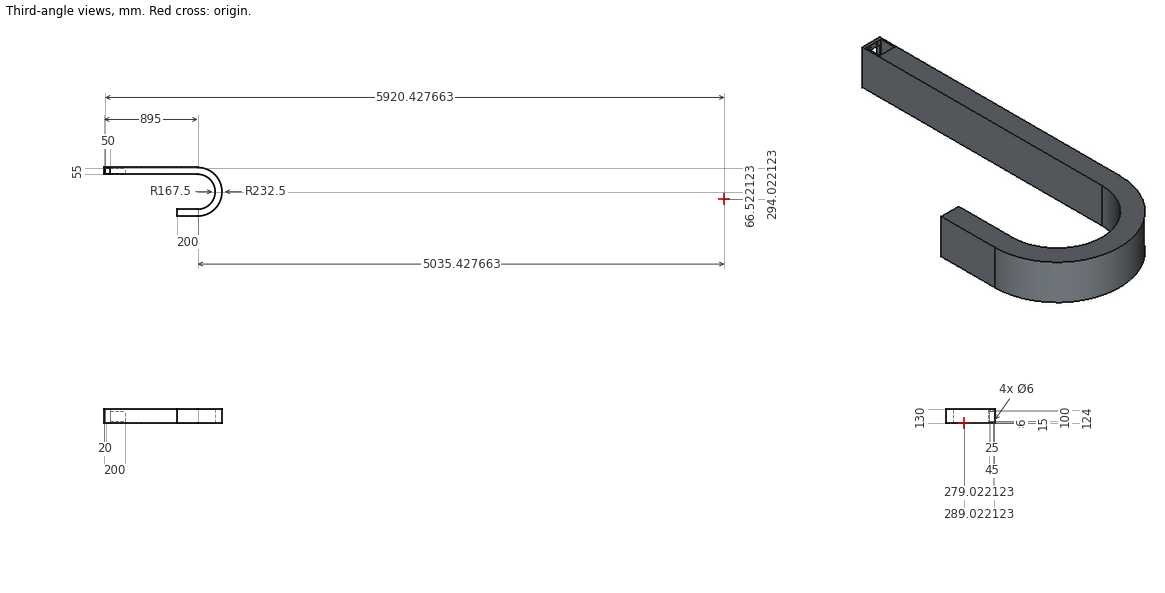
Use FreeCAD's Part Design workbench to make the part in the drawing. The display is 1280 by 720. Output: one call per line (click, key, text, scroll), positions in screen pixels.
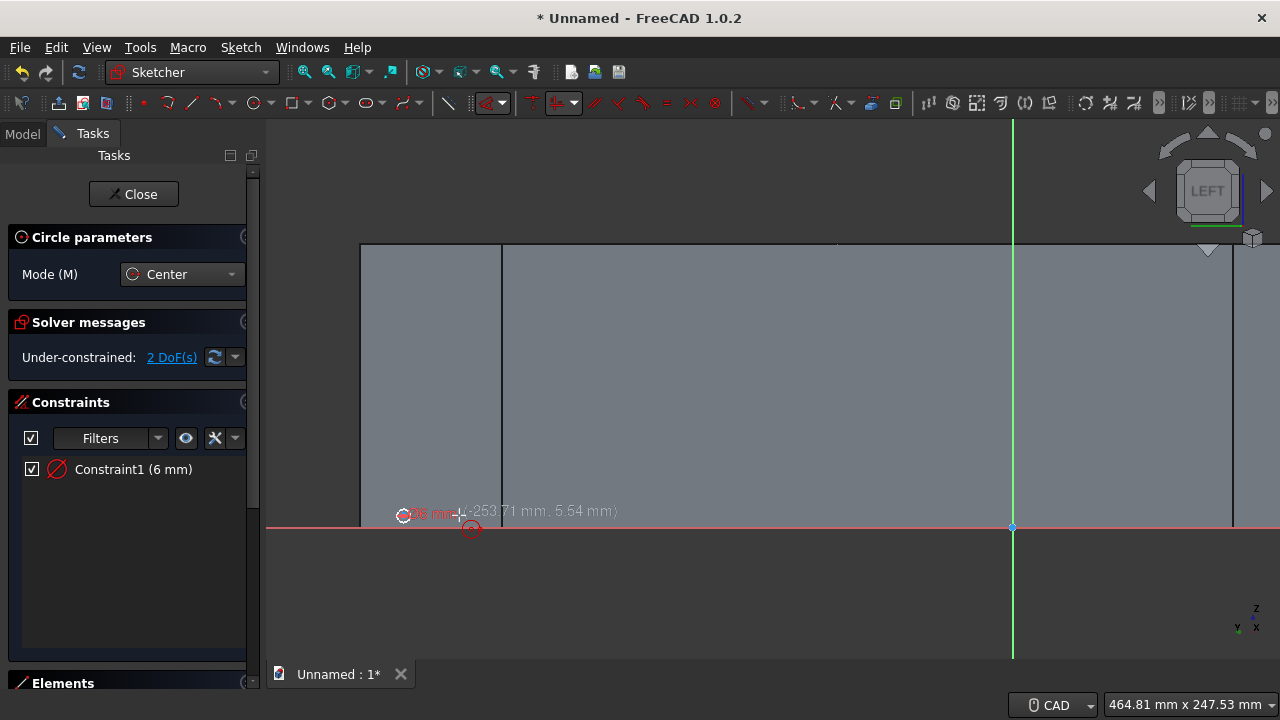
click(458, 515)
move(463, 510)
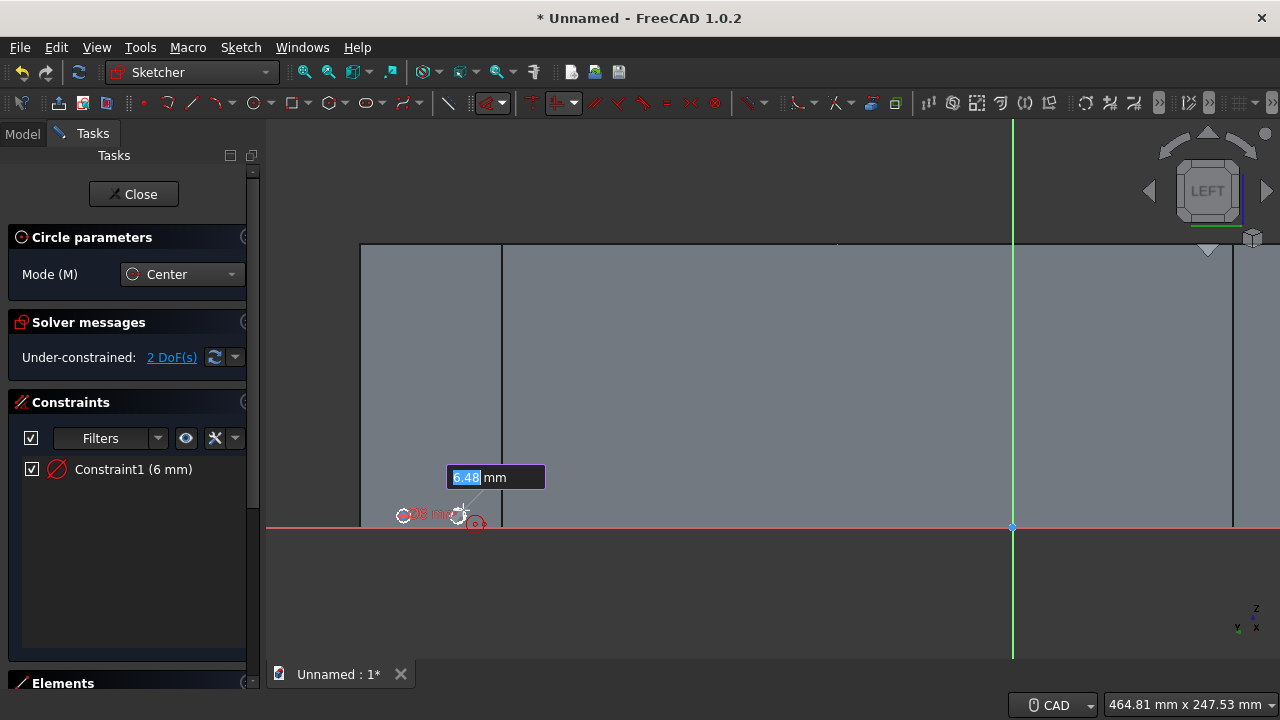
text(6)
key(Return)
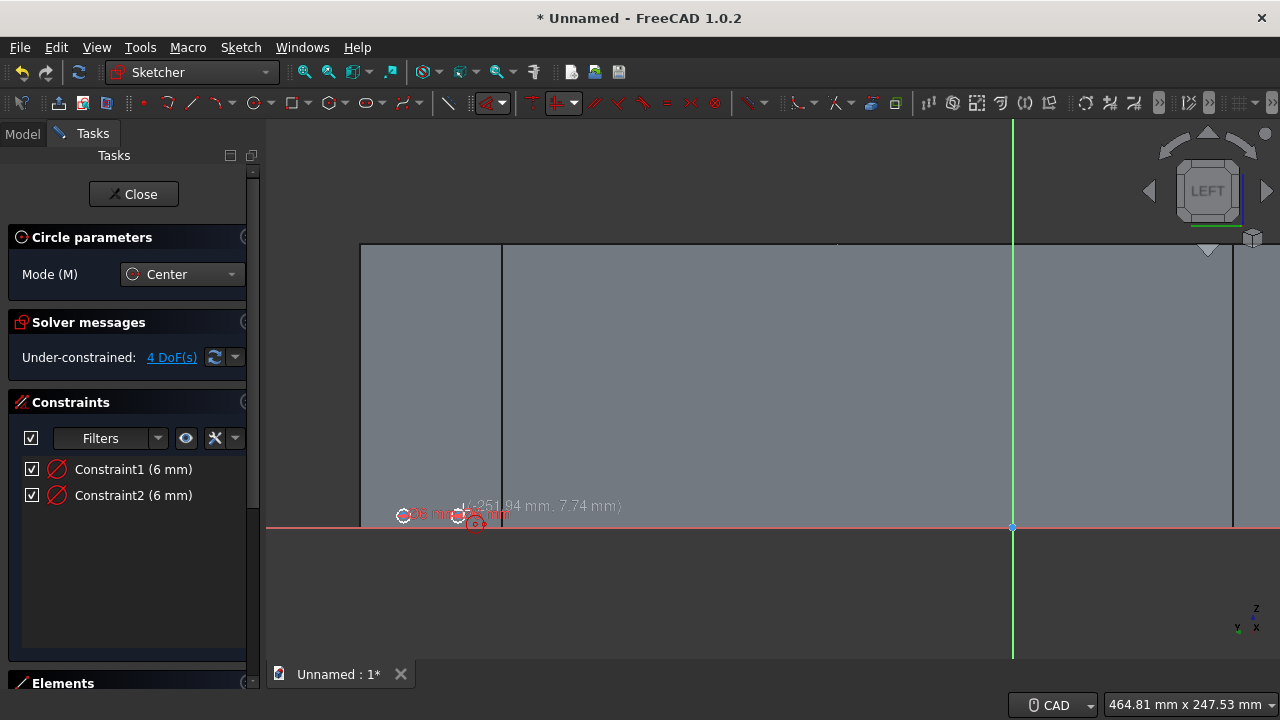
scroll(404, 257, up, 7)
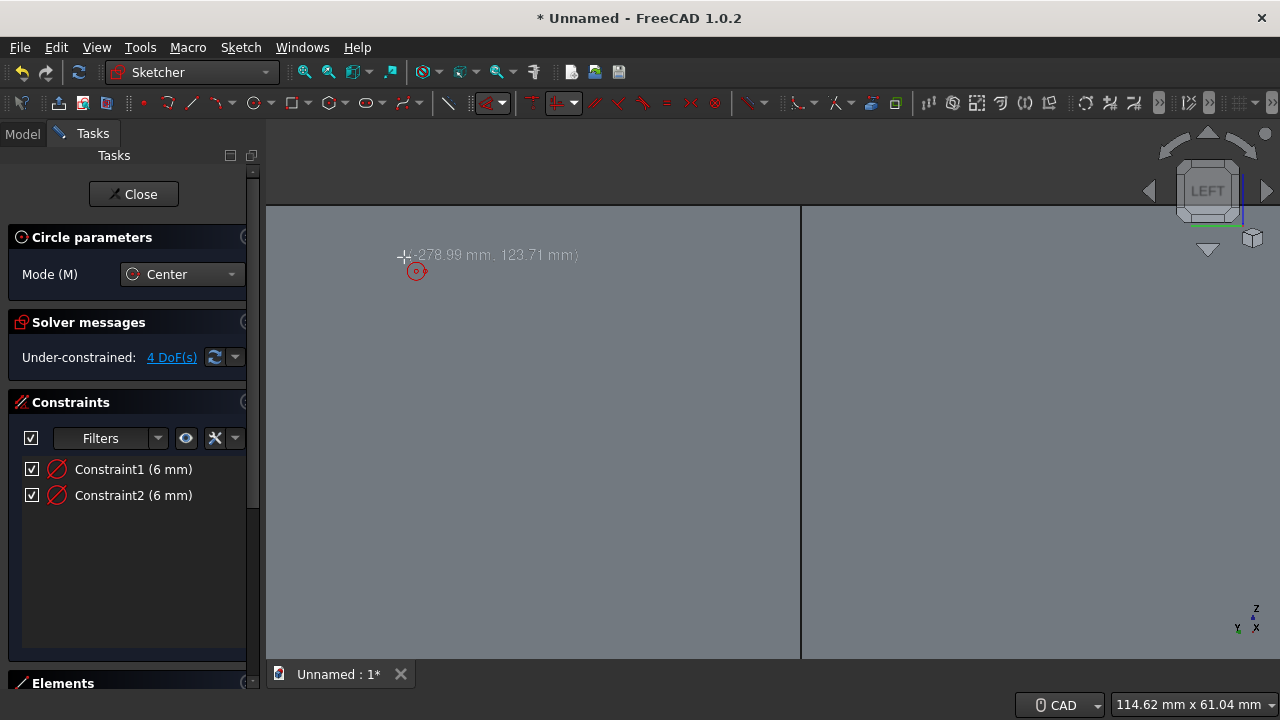
scroll(403, 257, down, 7)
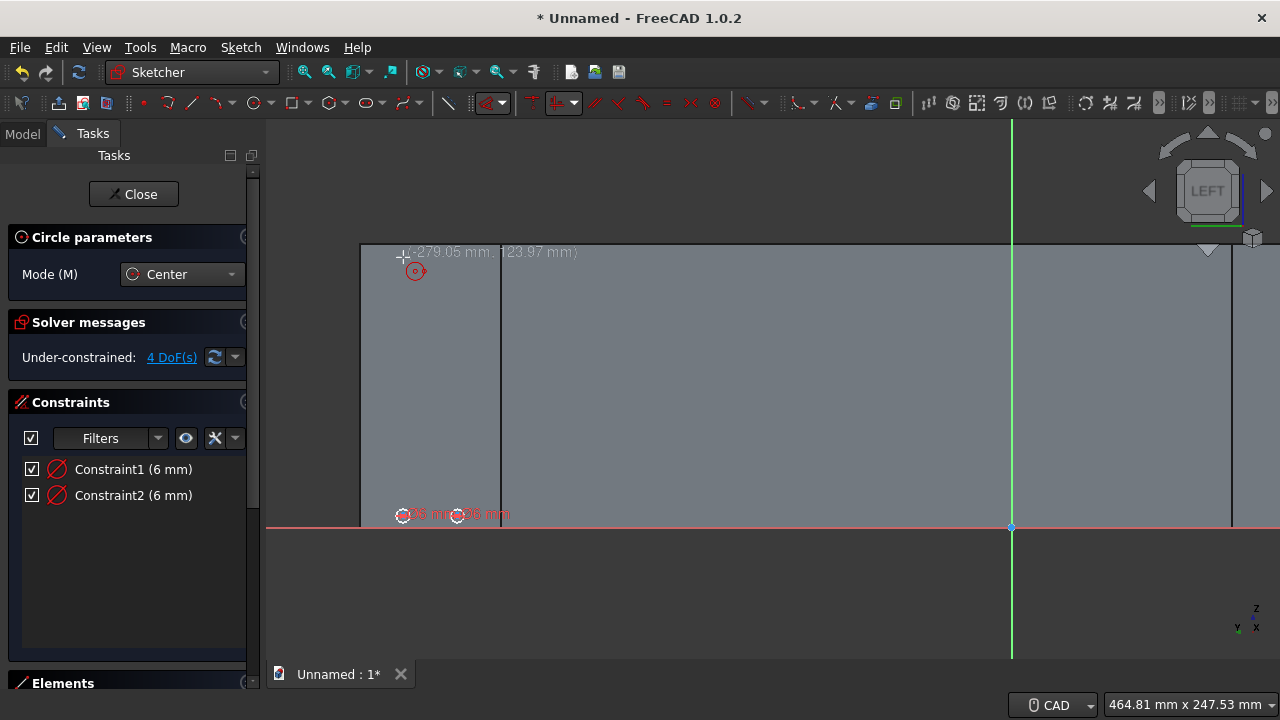
click(403, 257)
move(408, 253)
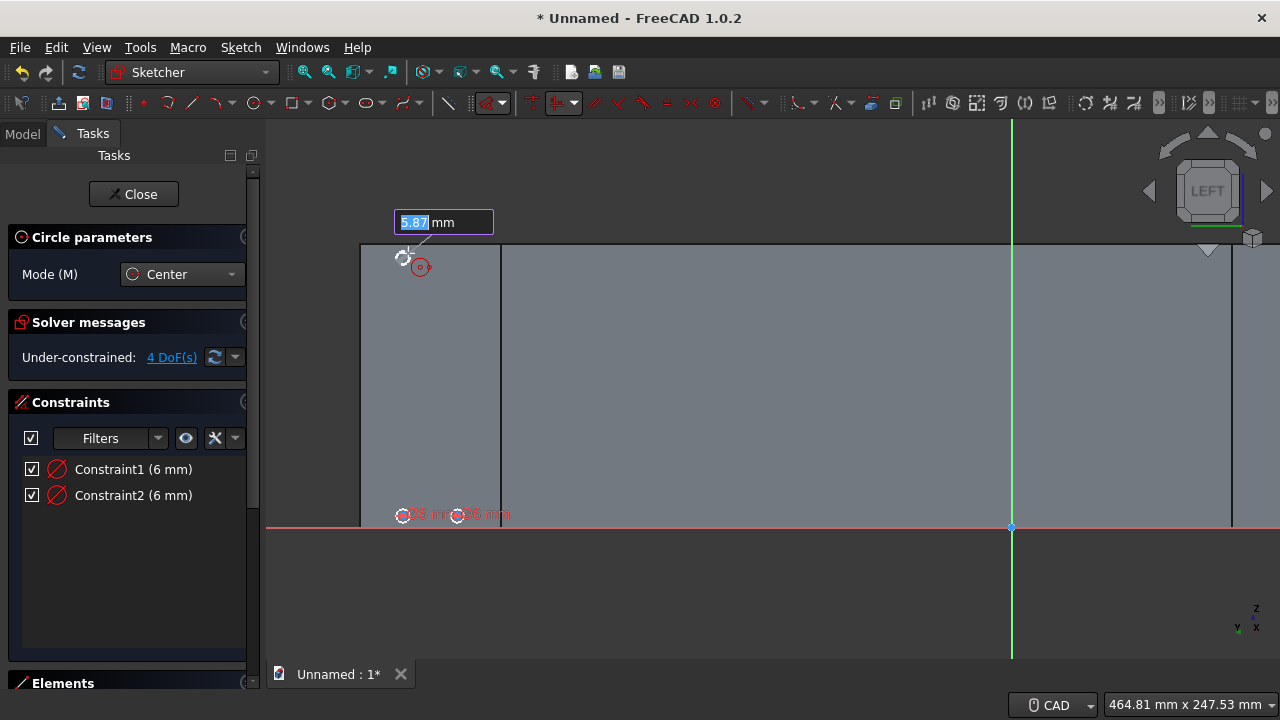
text(6)
key(Return)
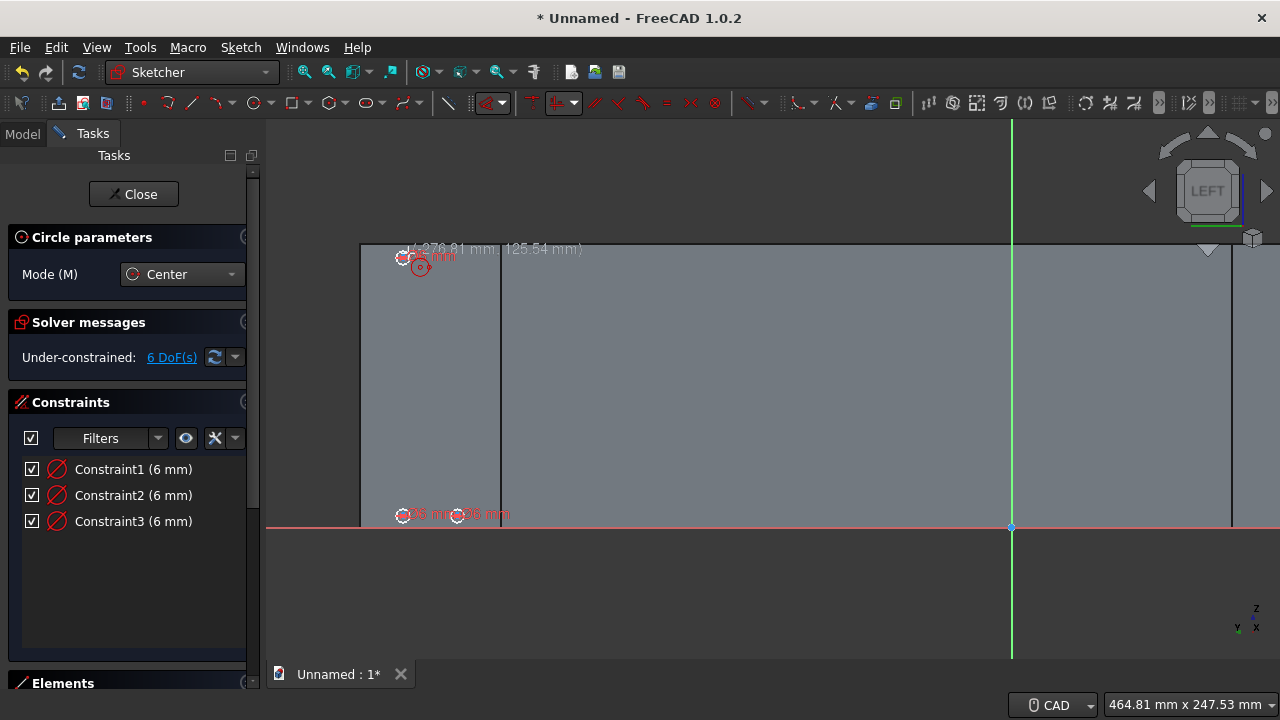
scroll(458, 257, up, 7)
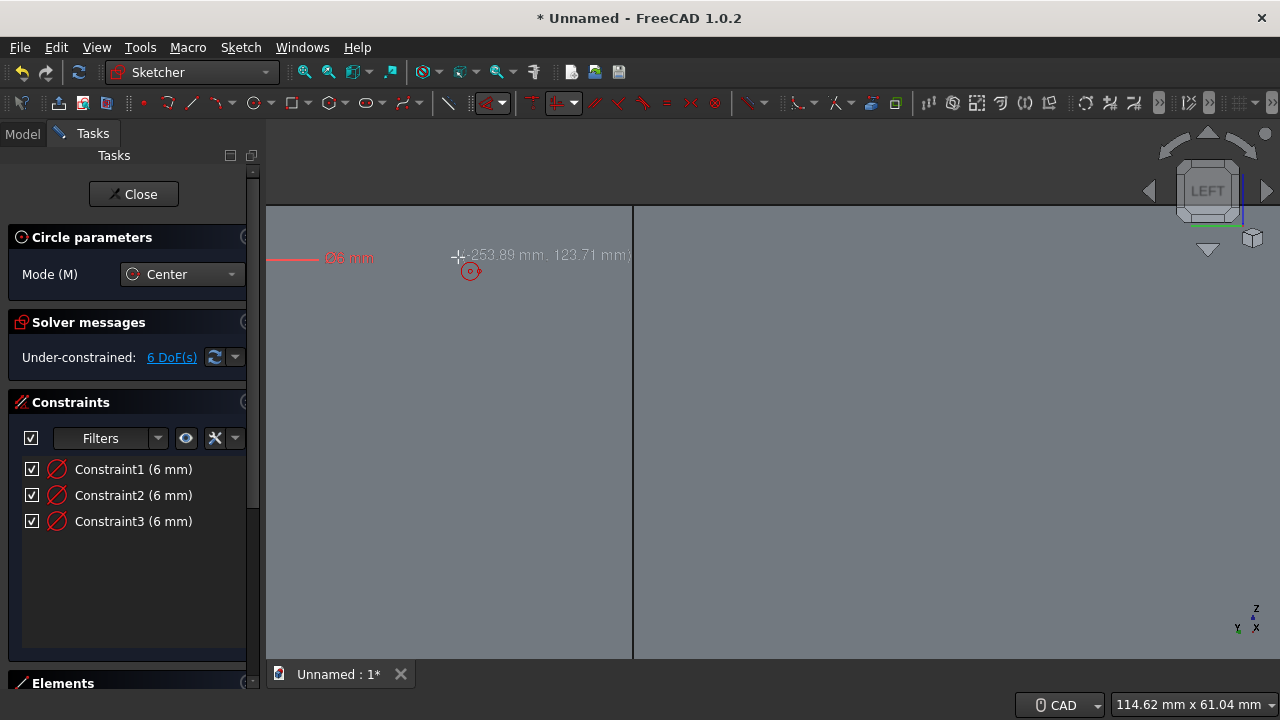
scroll(459, 257, down, 7)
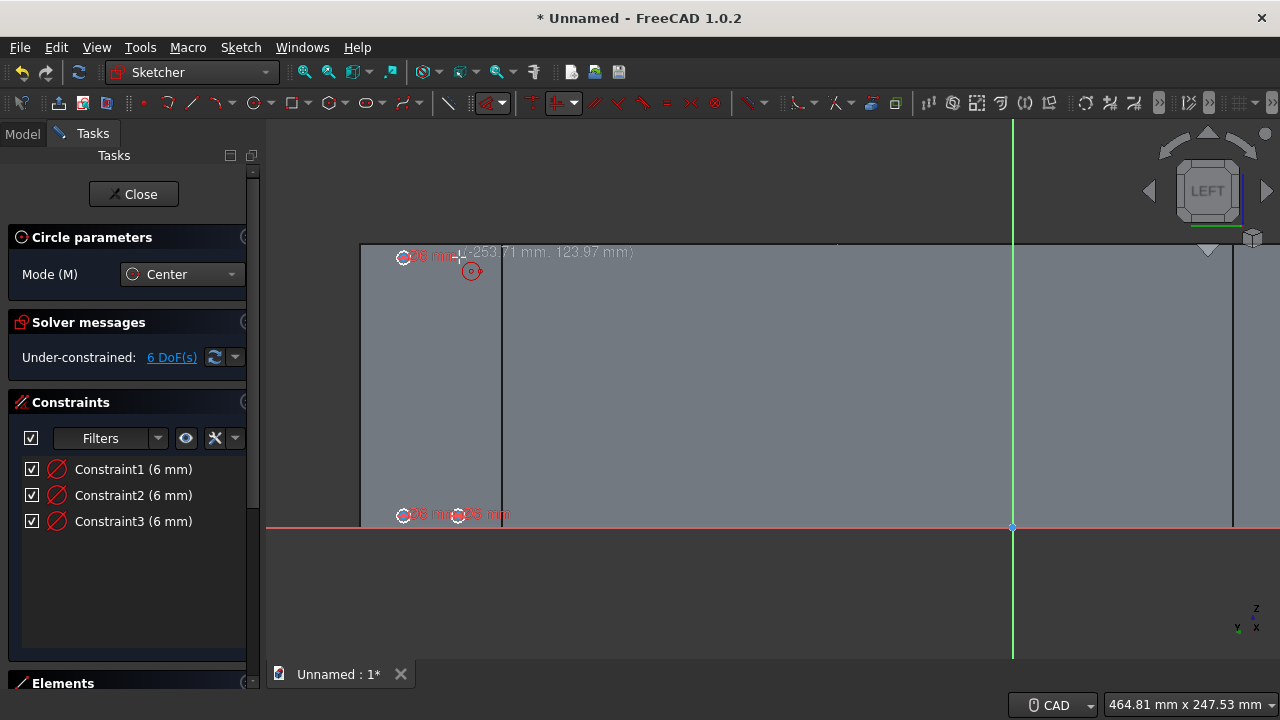
click(458, 257)
move(463, 253)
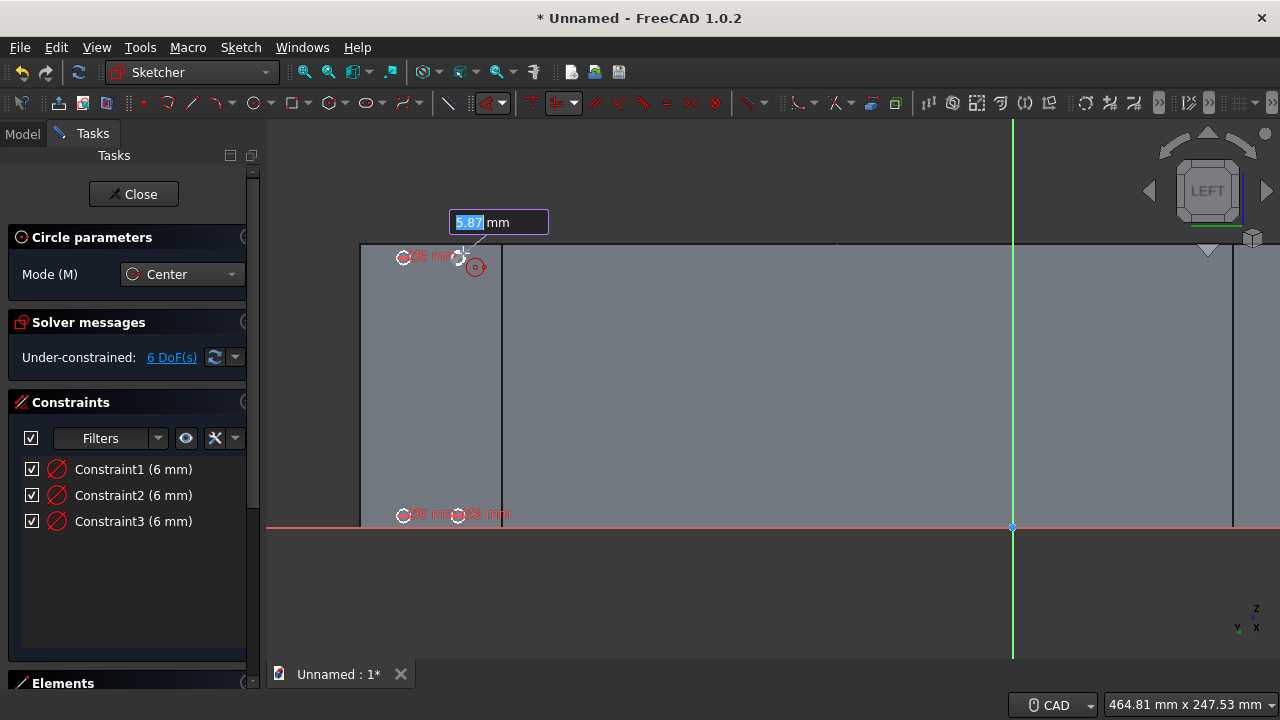
text(6)
key(Return)
key(Escape)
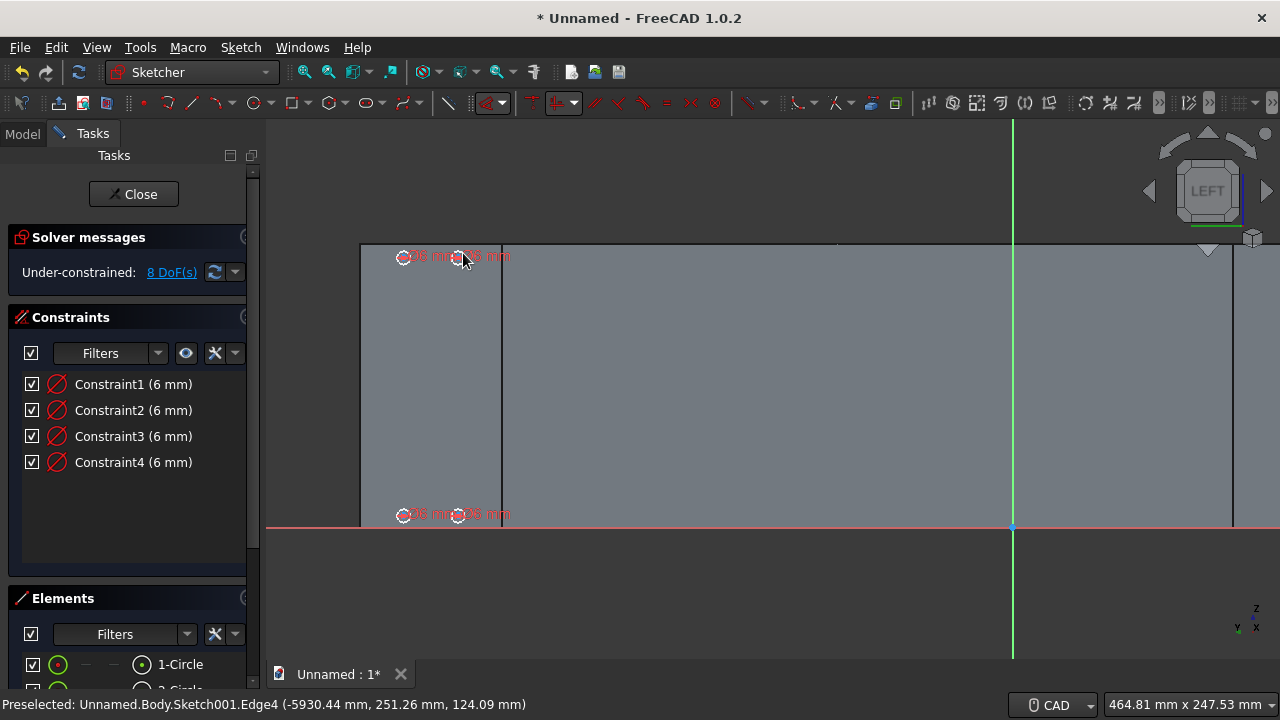
click(404, 516)